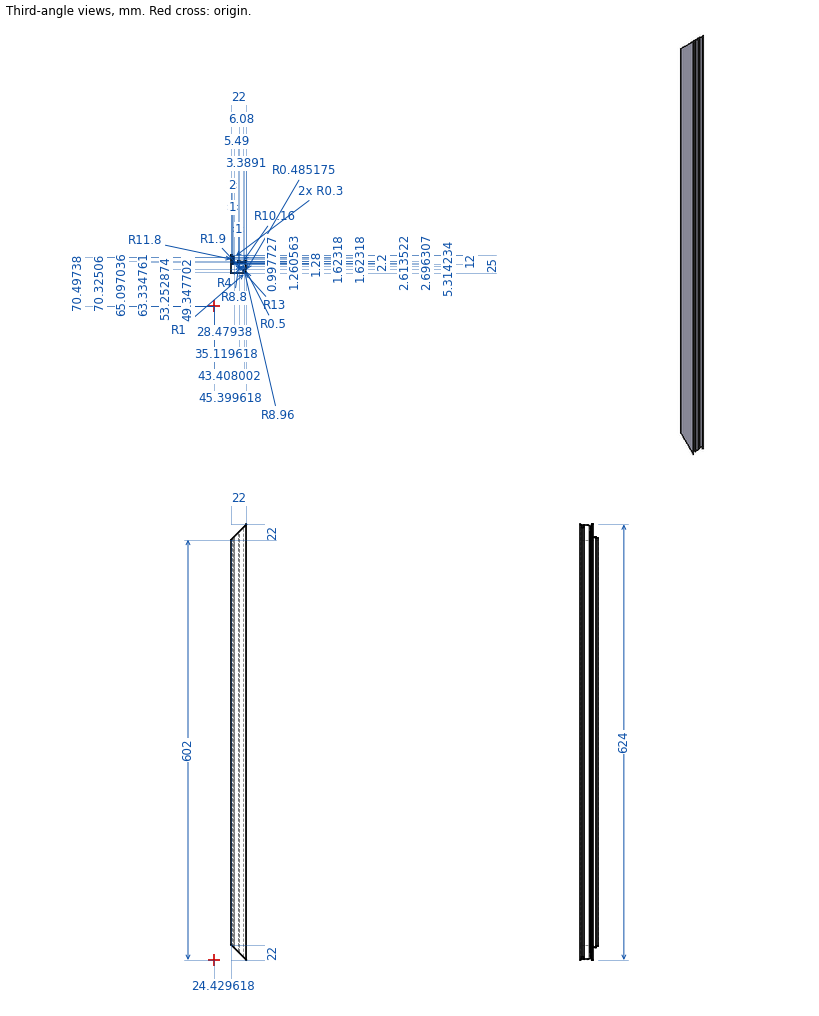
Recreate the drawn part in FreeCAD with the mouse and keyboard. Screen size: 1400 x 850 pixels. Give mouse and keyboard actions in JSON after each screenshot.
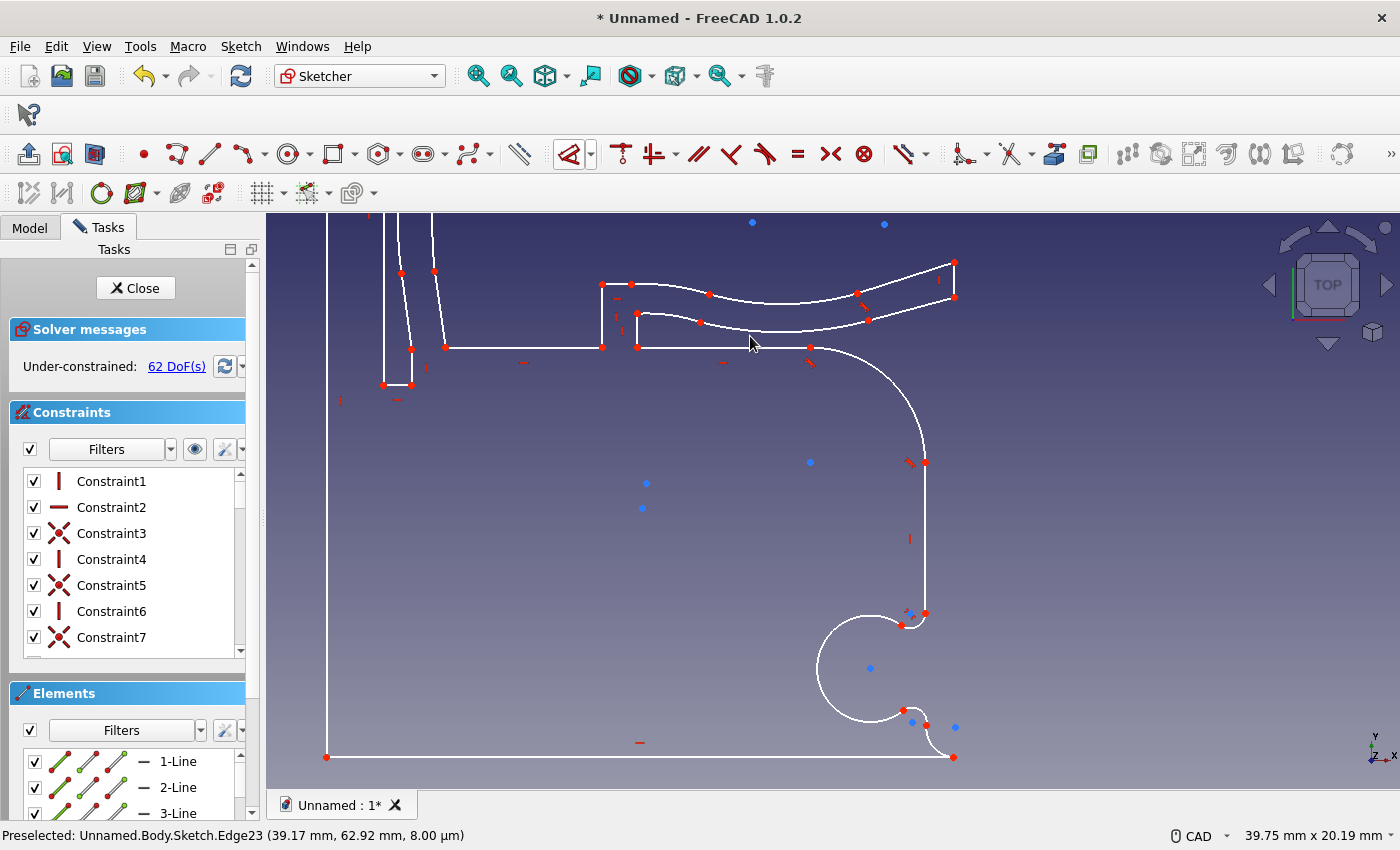
{"action": "left_click", "coordinate": [925, 272]}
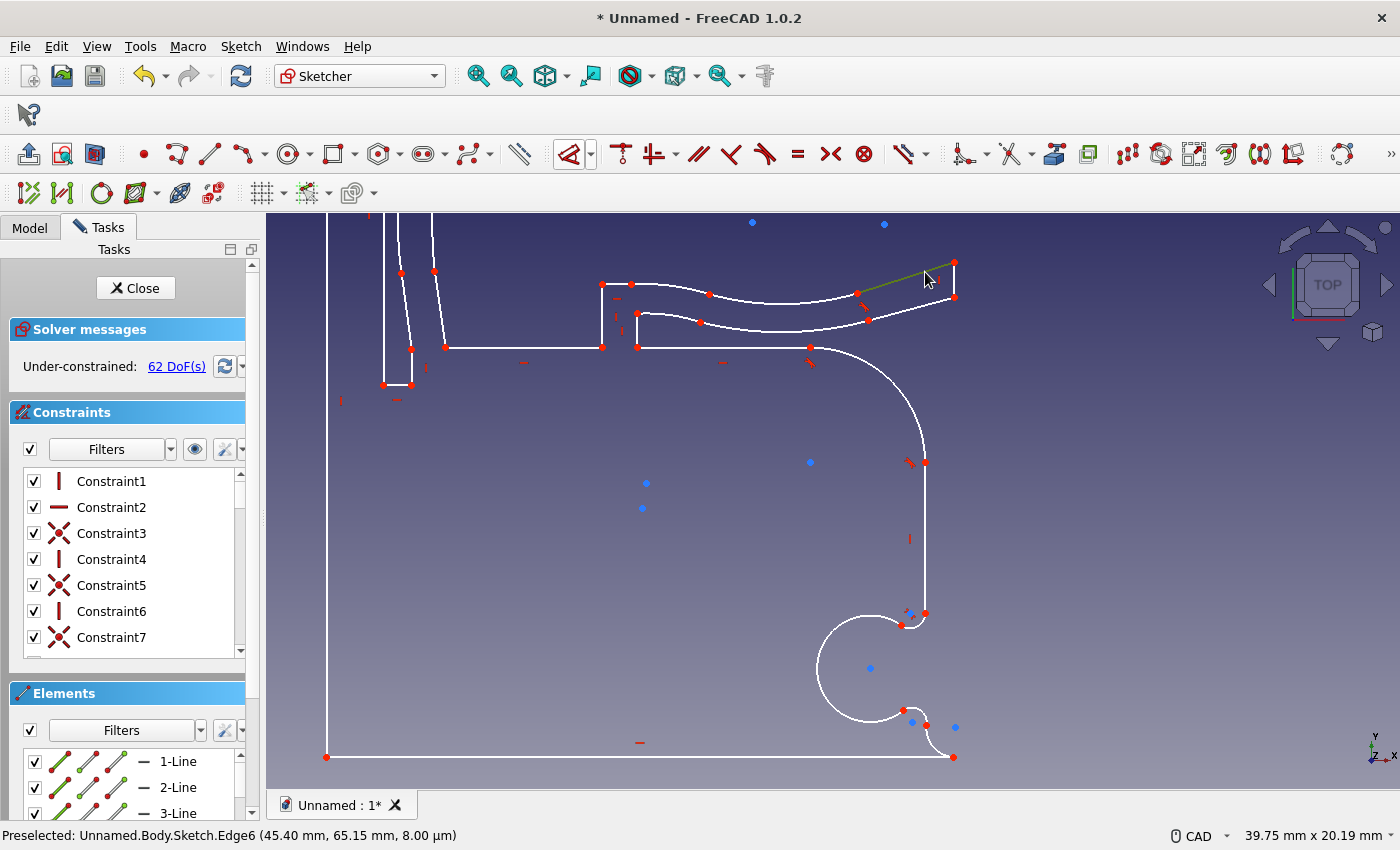
{"action": "left_click", "coordinate": [754, 303]}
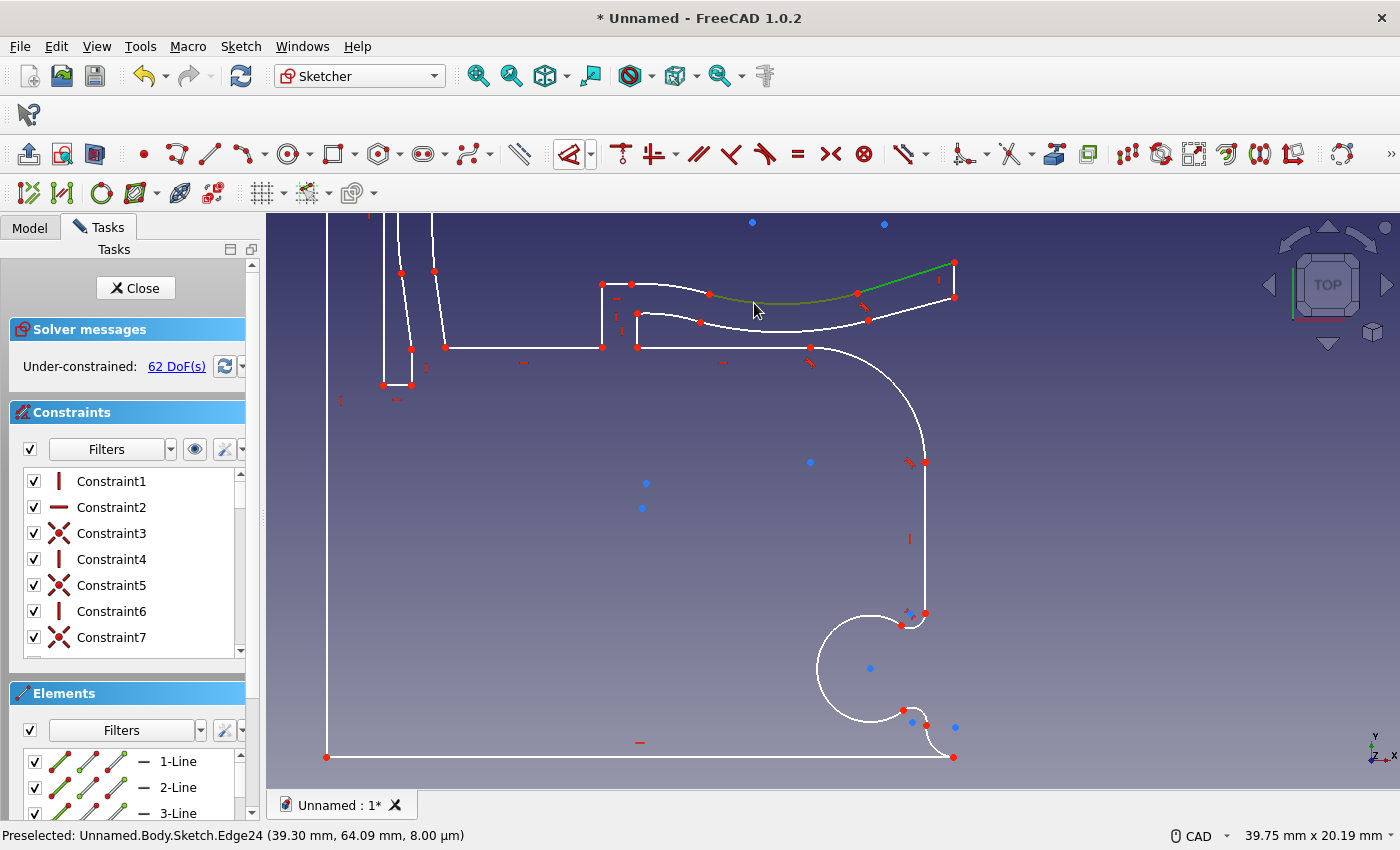
{"action": "left_click", "coordinate": [765, 154]}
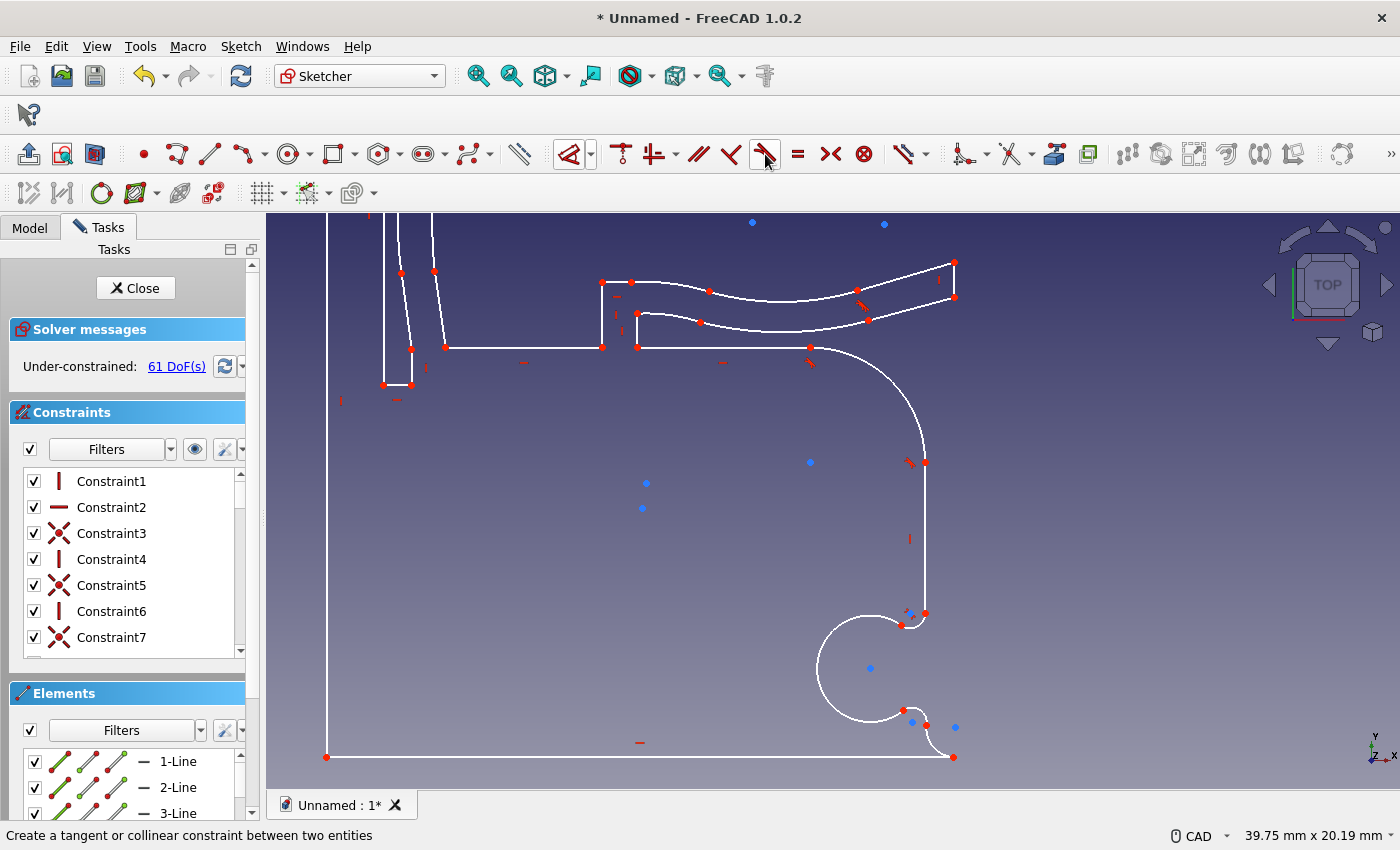
{"action": "left_click", "coordinate": [620, 282]}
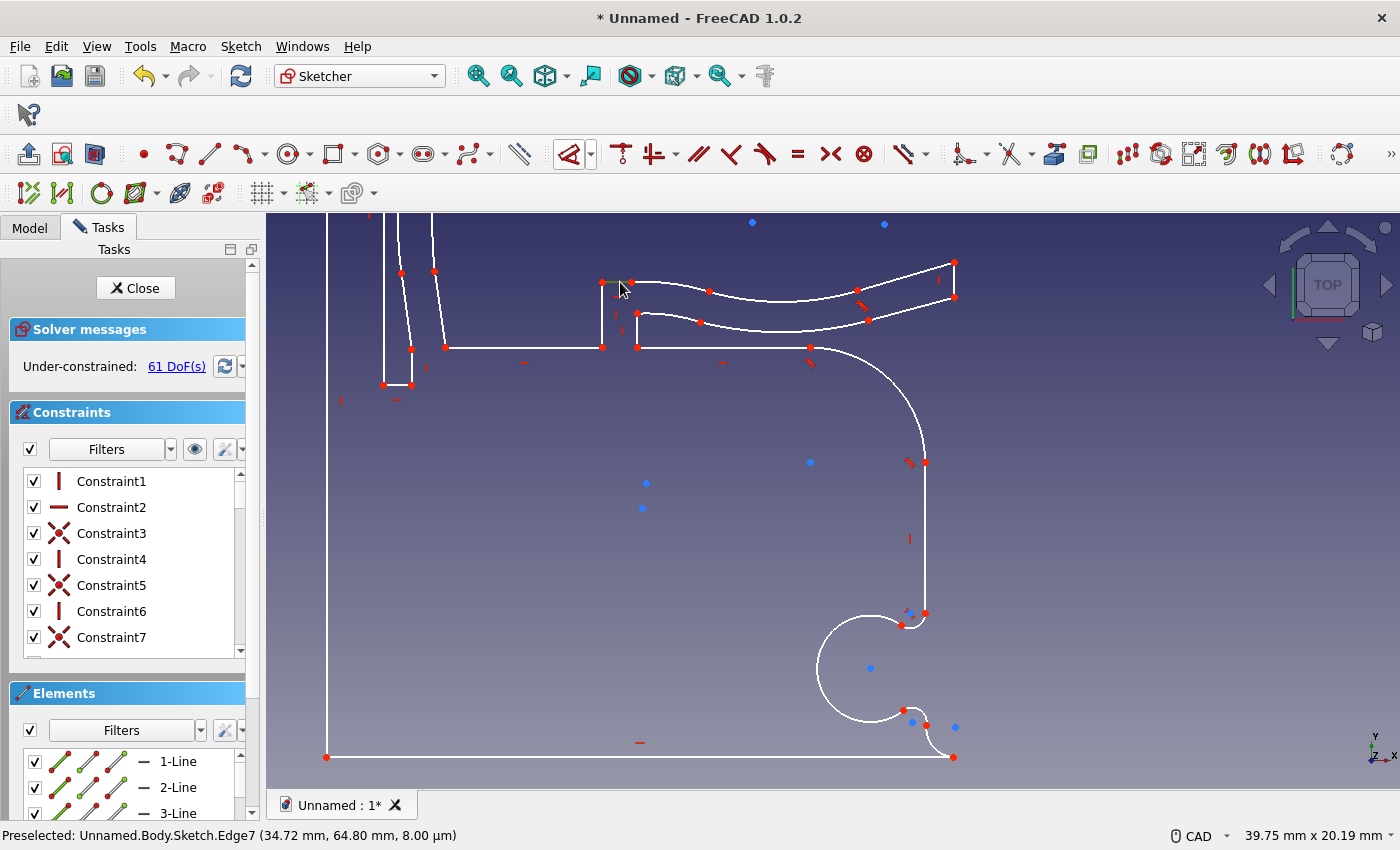
{"action": "left_click", "coordinate": [687, 286]}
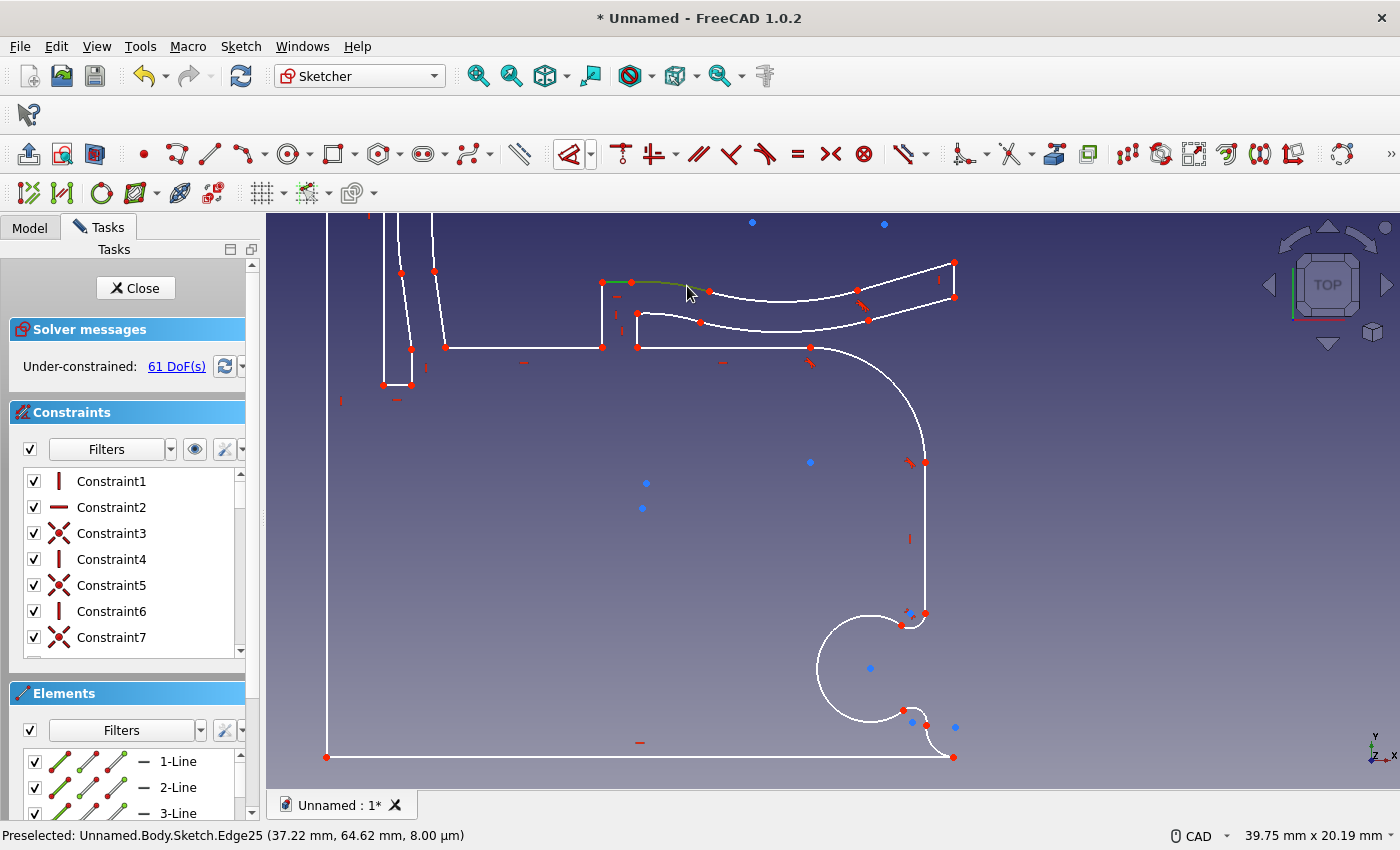
{"action": "key", "text": "t"}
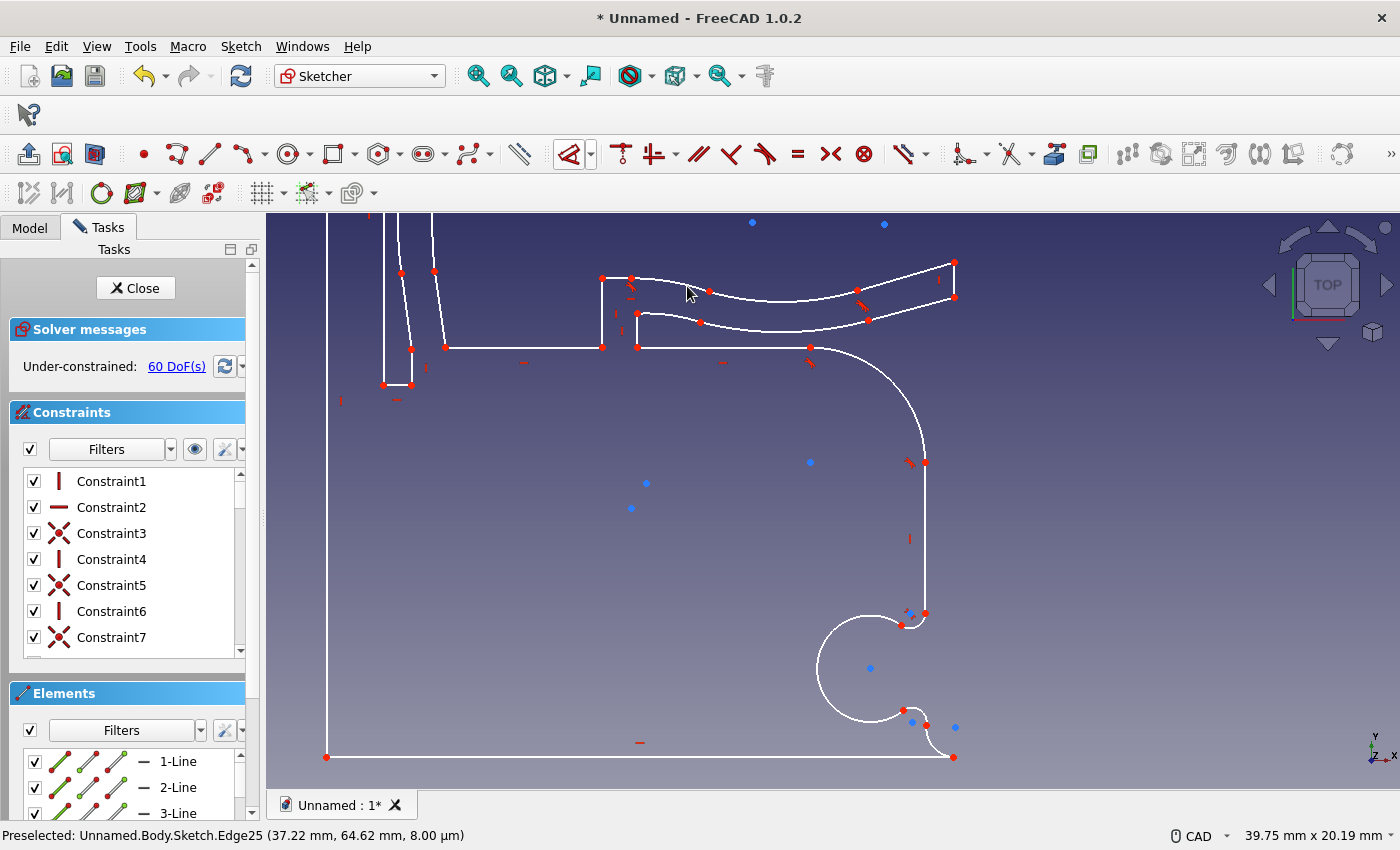
{"action": "left_click", "coordinate": [442, 325]}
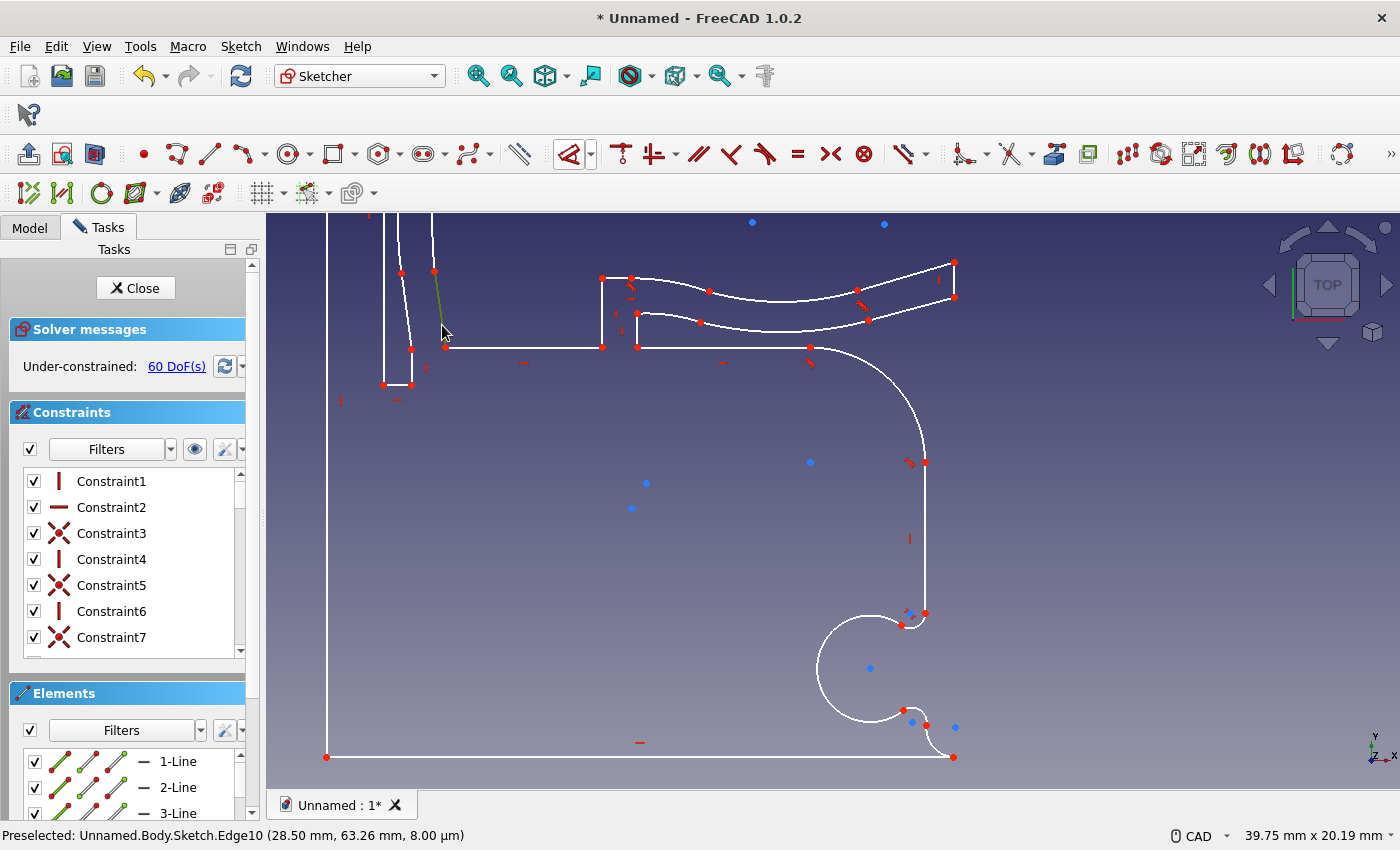
{"action": "left_click", "coordinate": [433, 243]}